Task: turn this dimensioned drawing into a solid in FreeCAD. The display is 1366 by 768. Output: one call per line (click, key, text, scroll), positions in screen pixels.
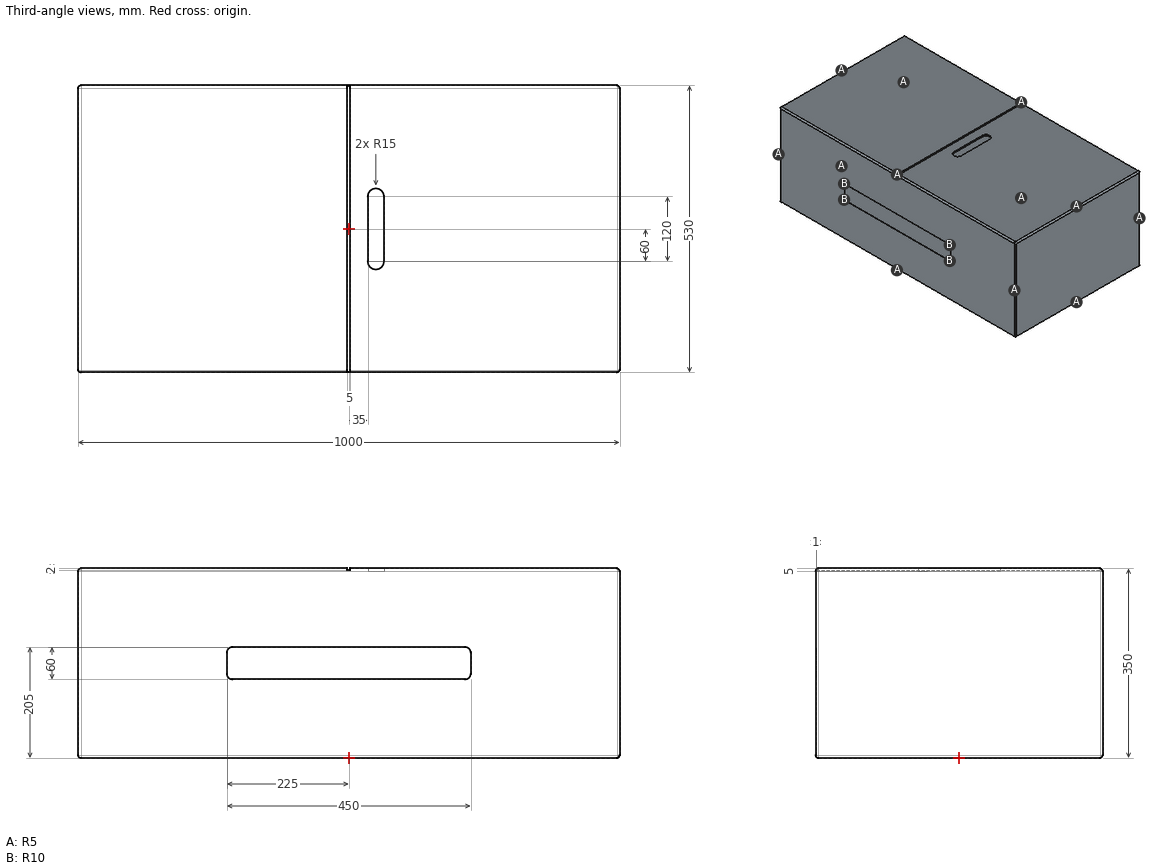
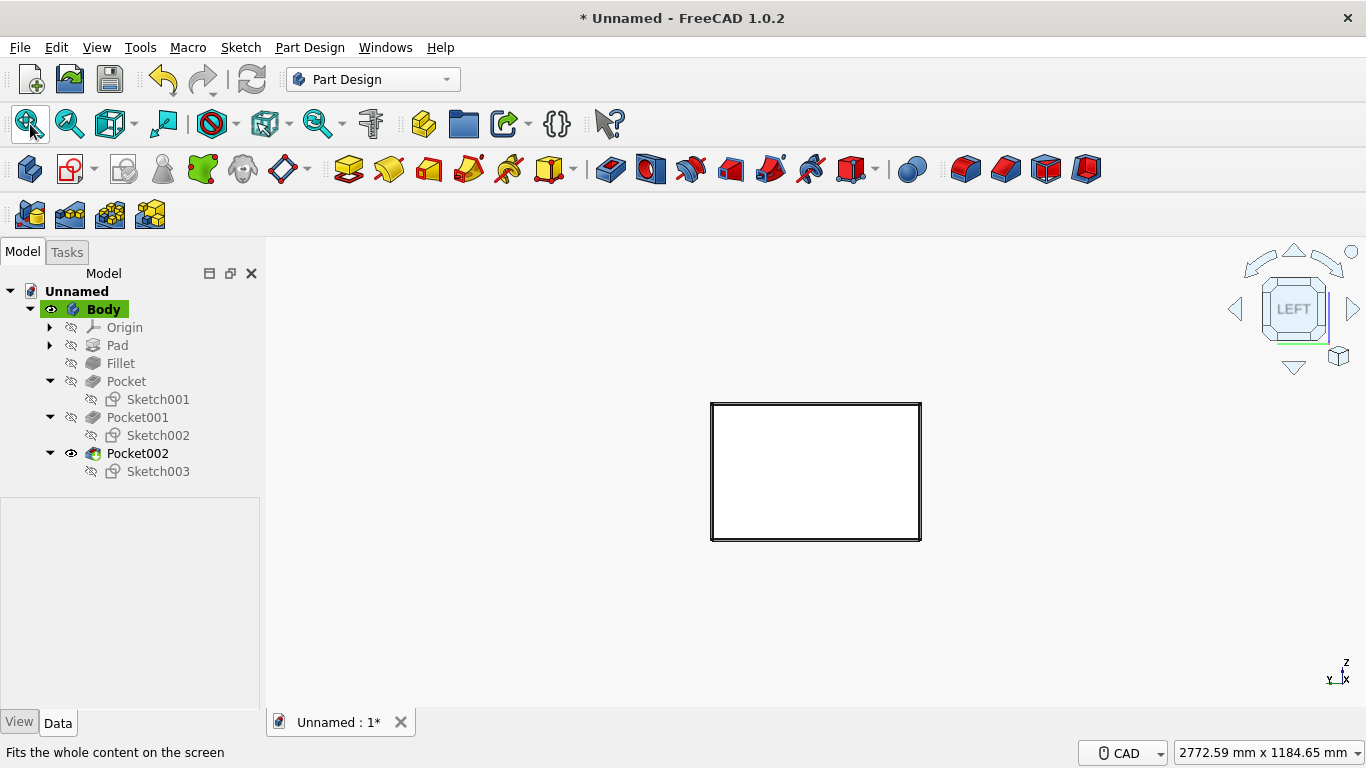
click(30, 124)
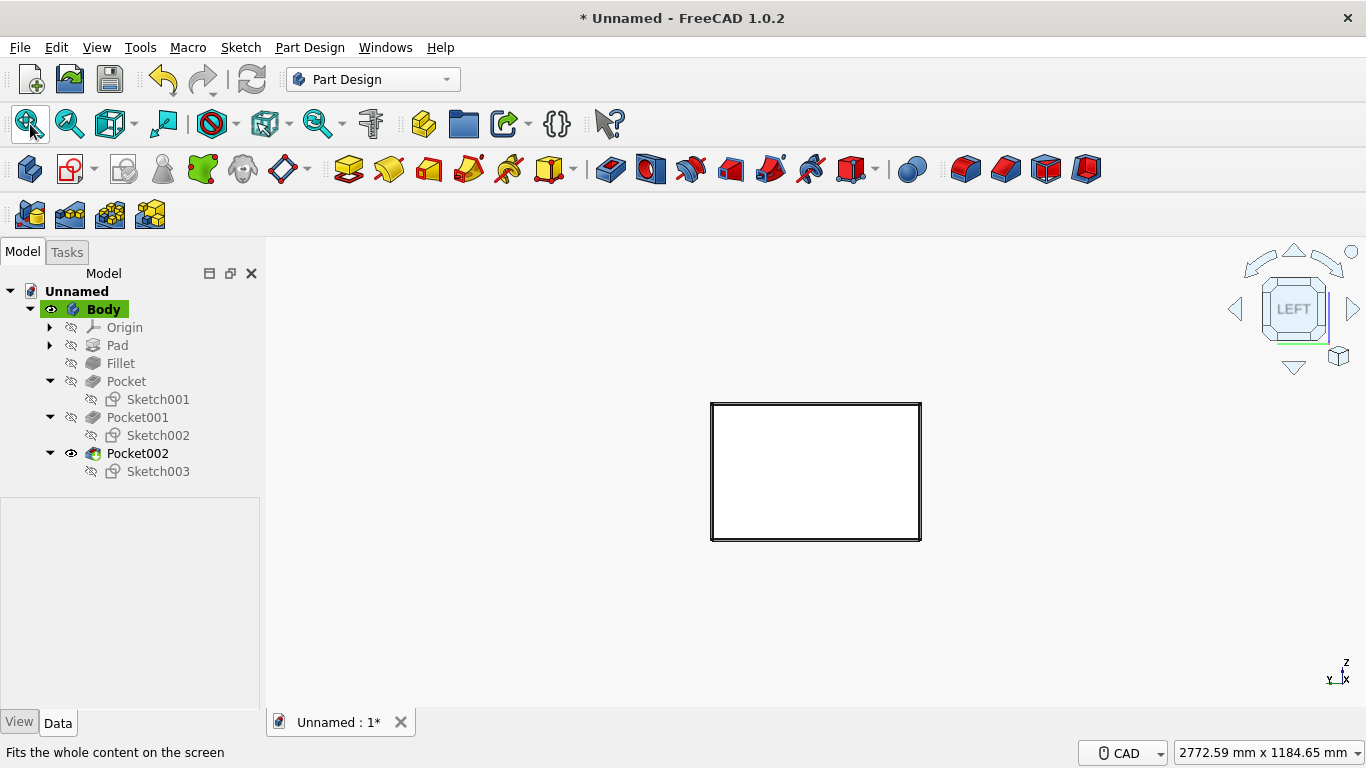
scroll(921, 459, up, 15)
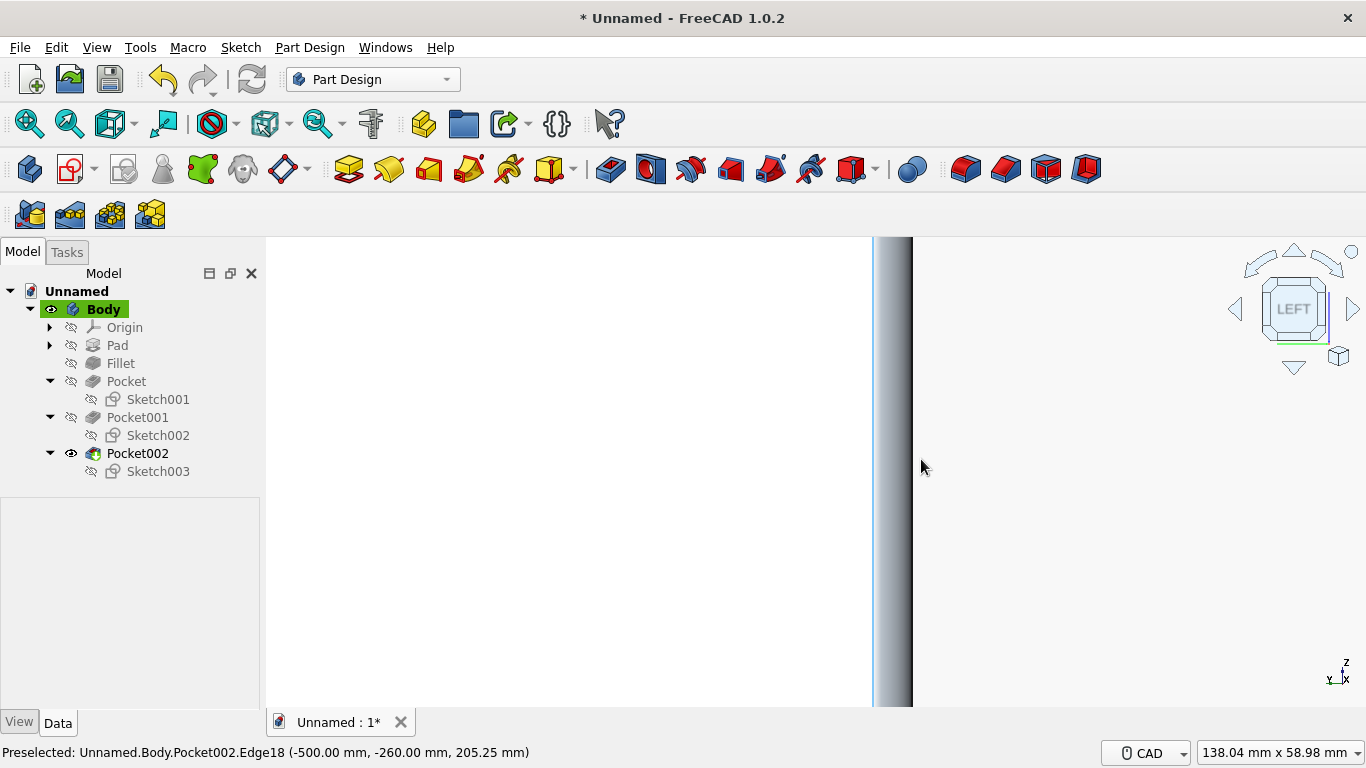
scroll(908, 471, up, 9)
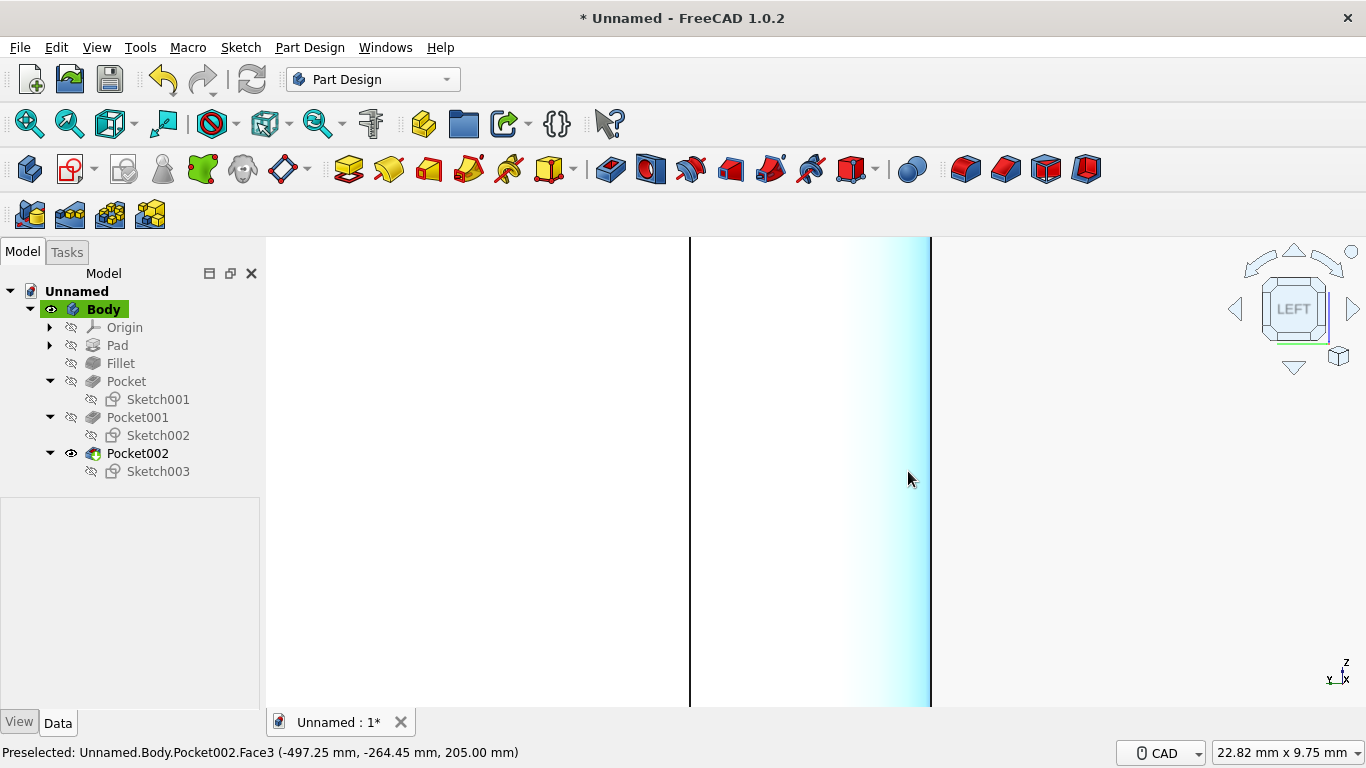
click(30, 124)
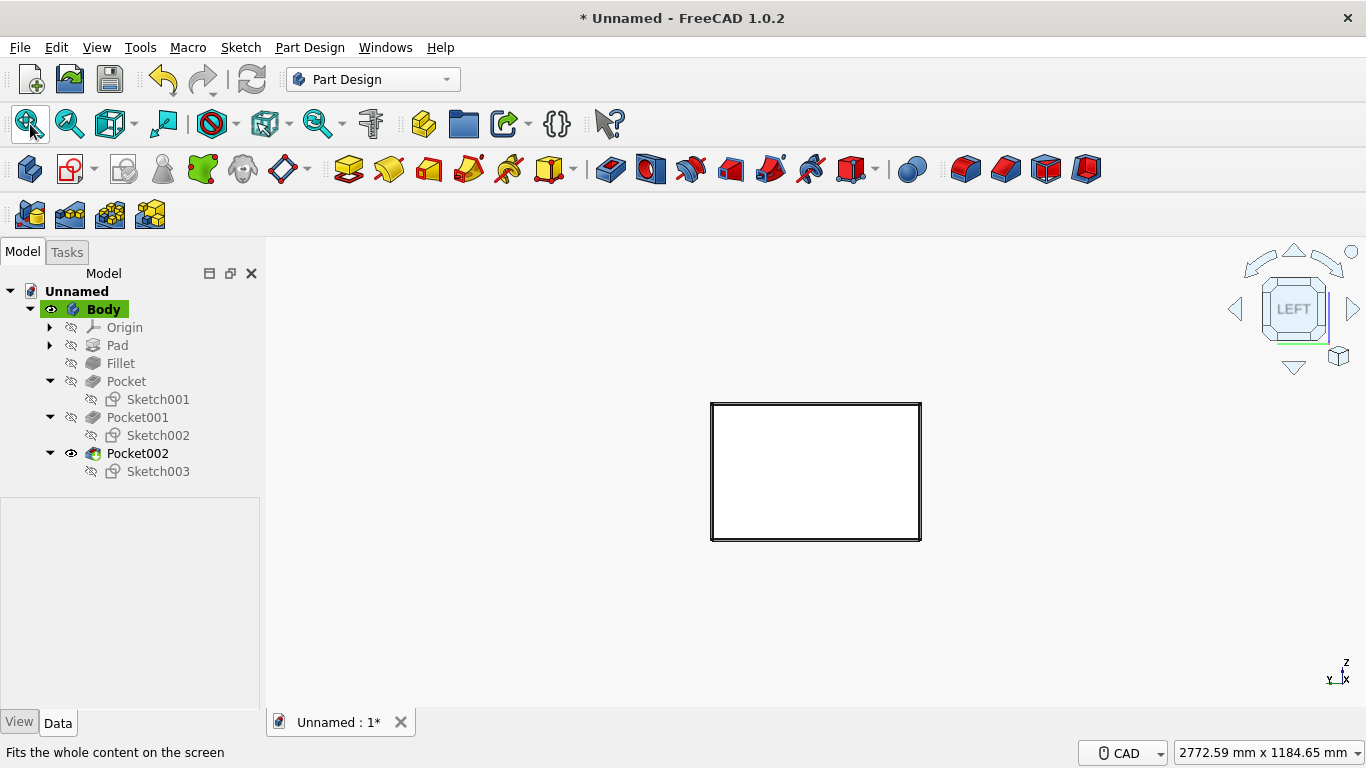
key(v)
key(3)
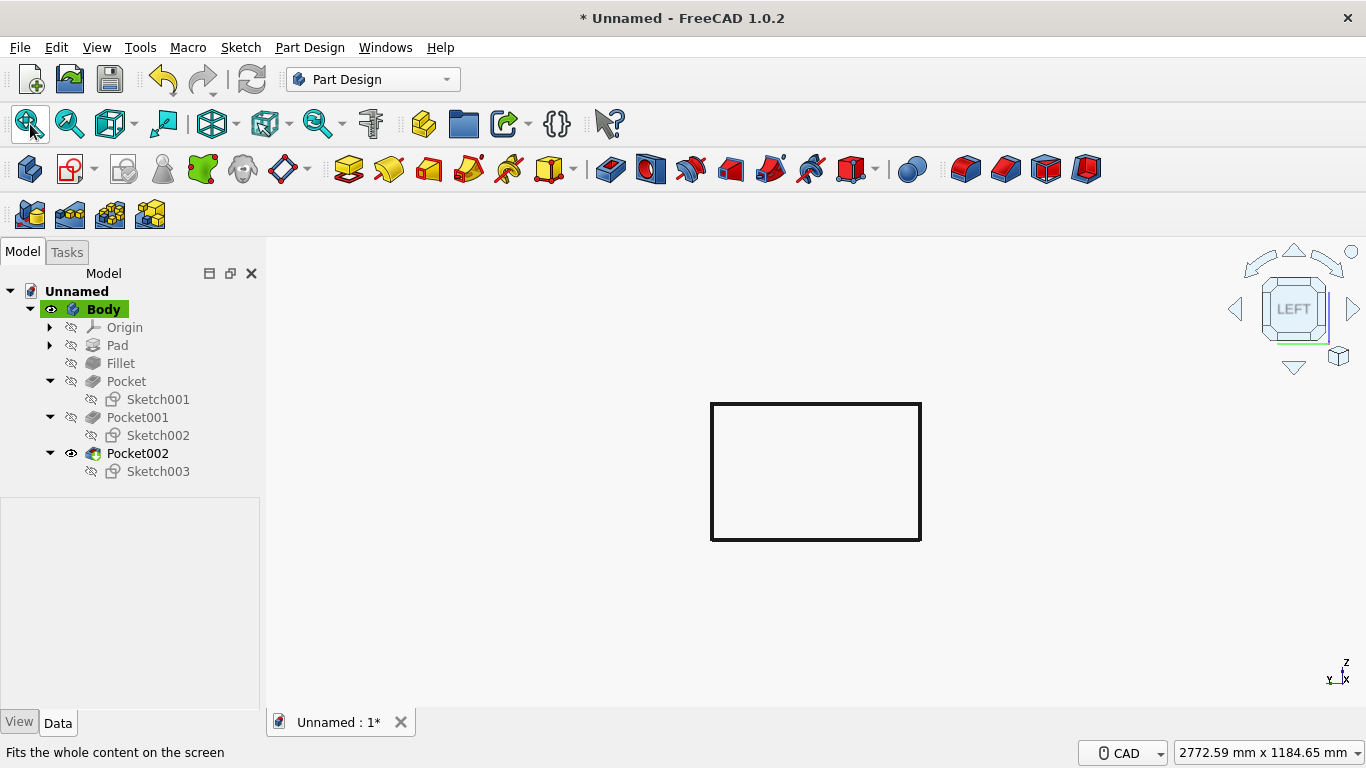
key(0)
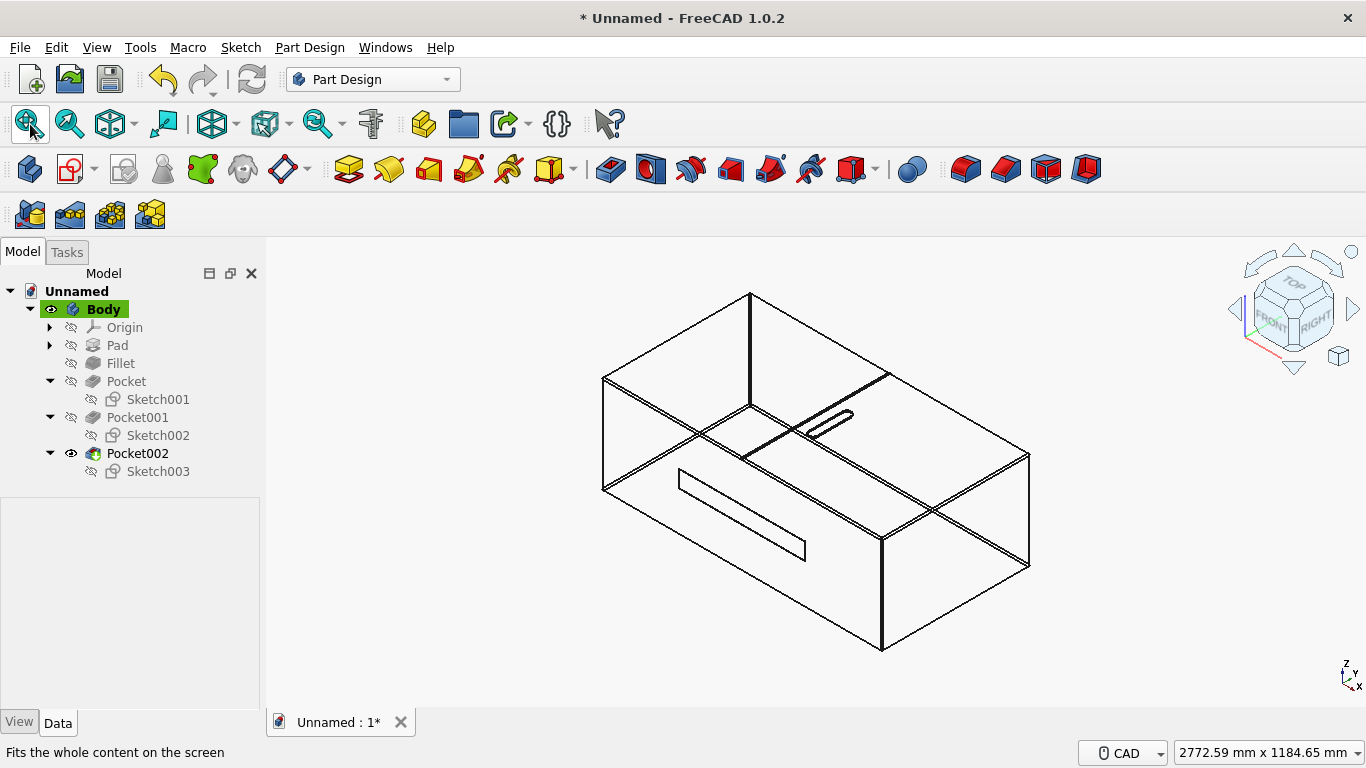
scroll(805, 541, up, 15)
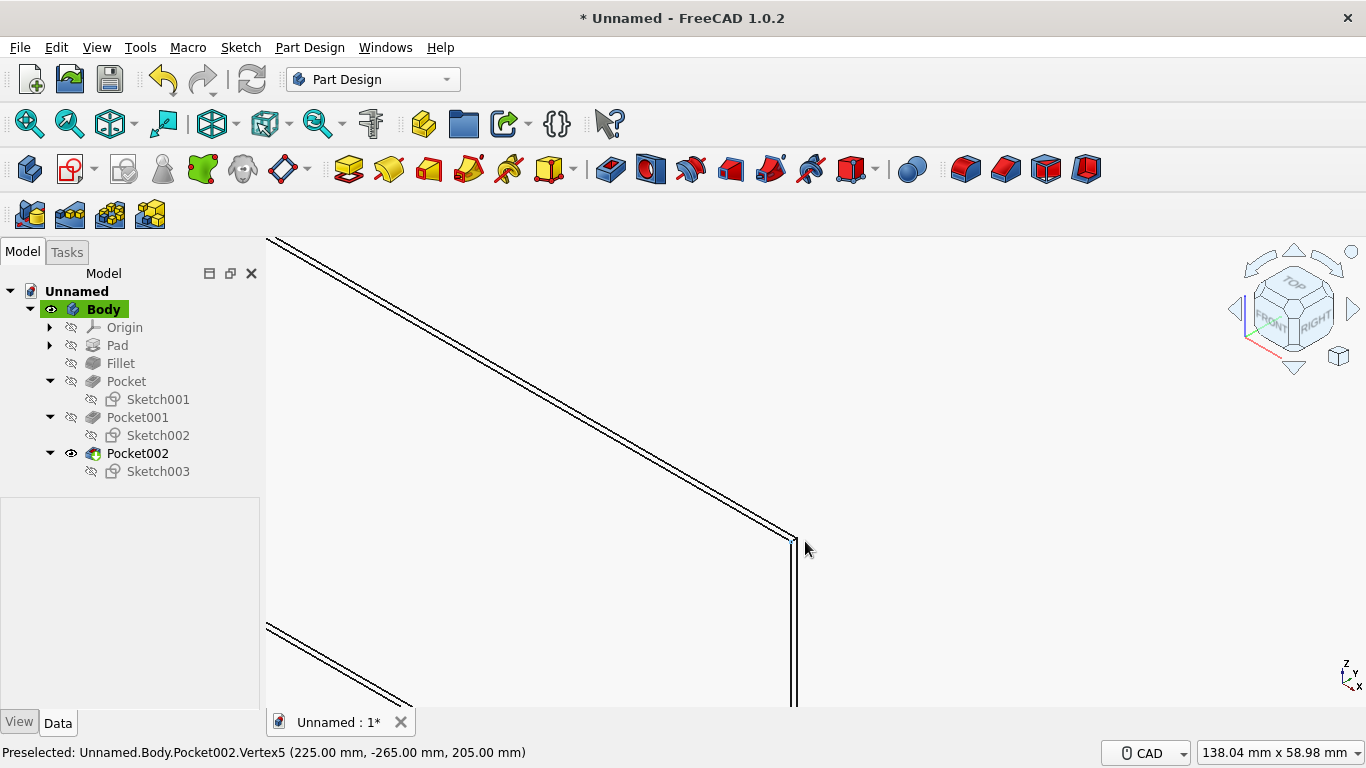
scroll(794, 539, up, 9)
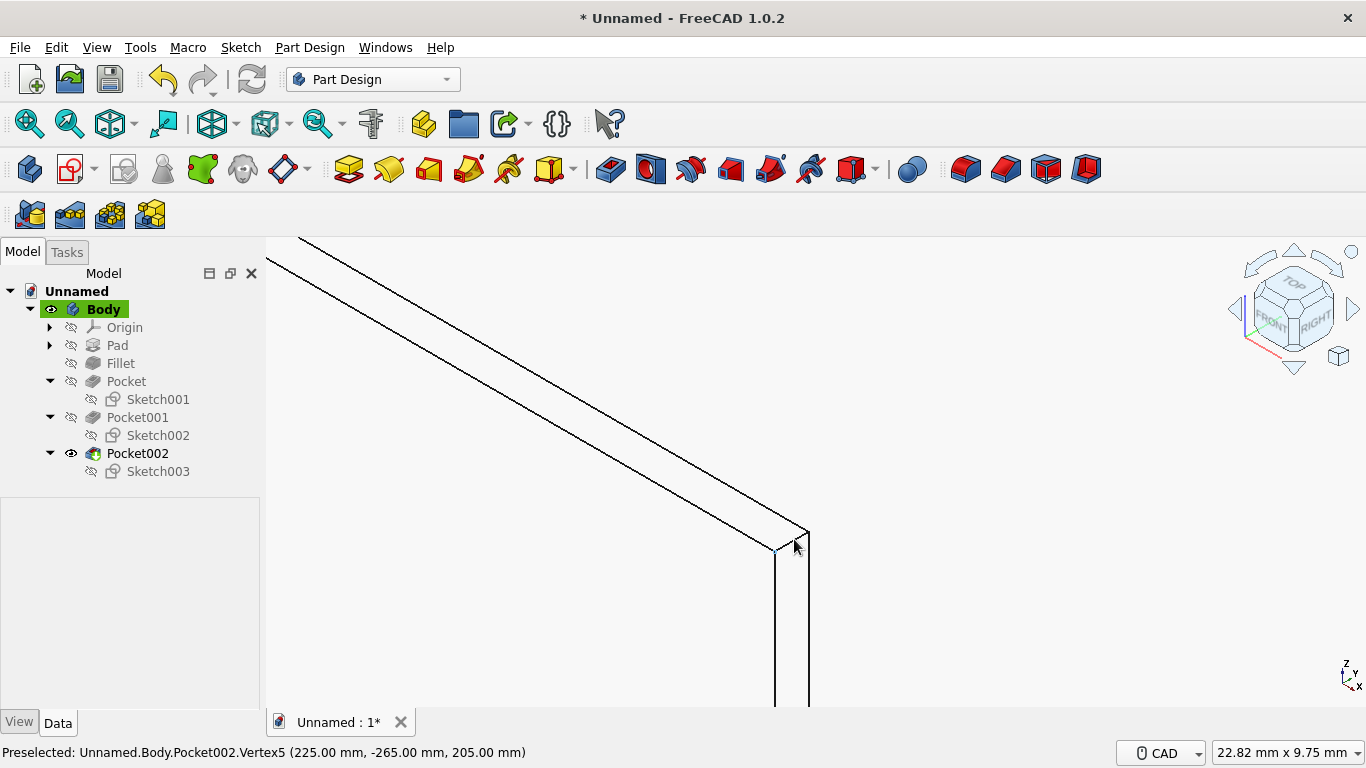
click(792, 541)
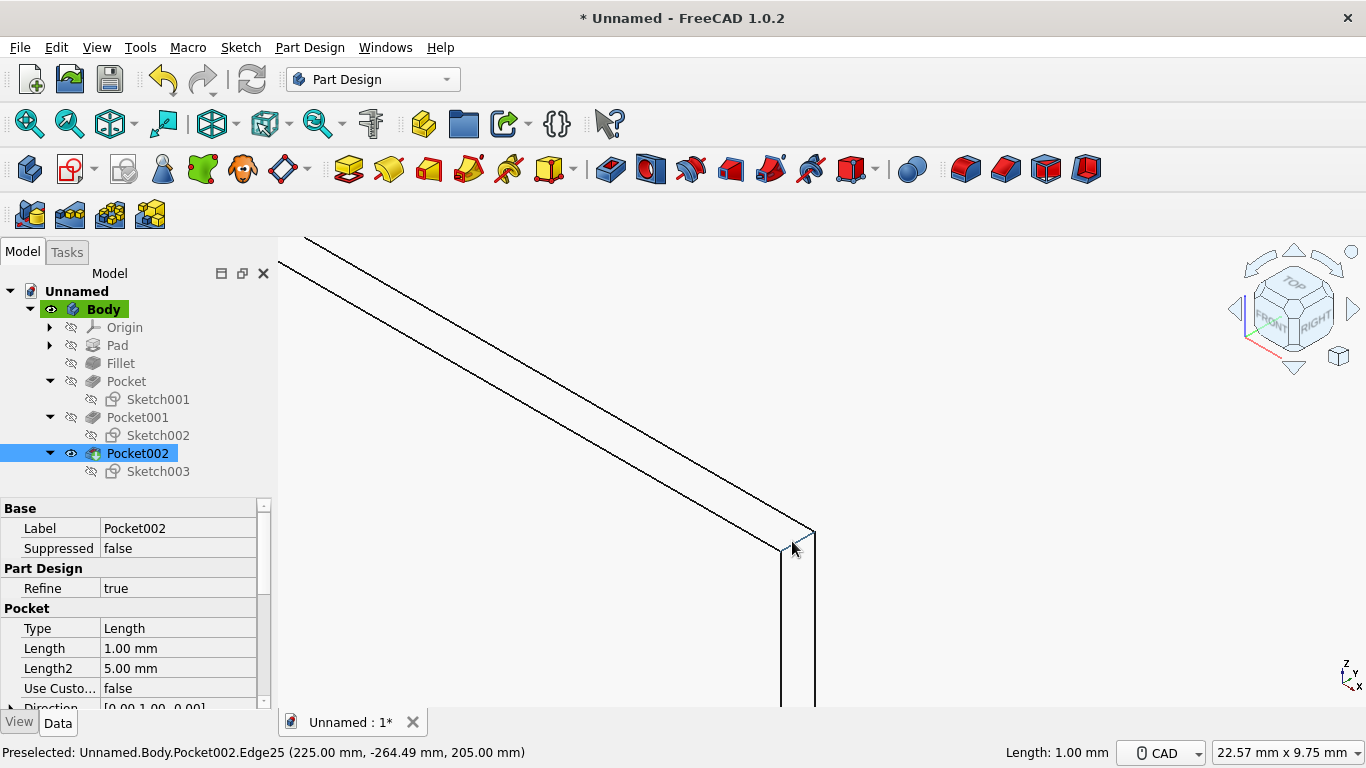
click(30, 124)